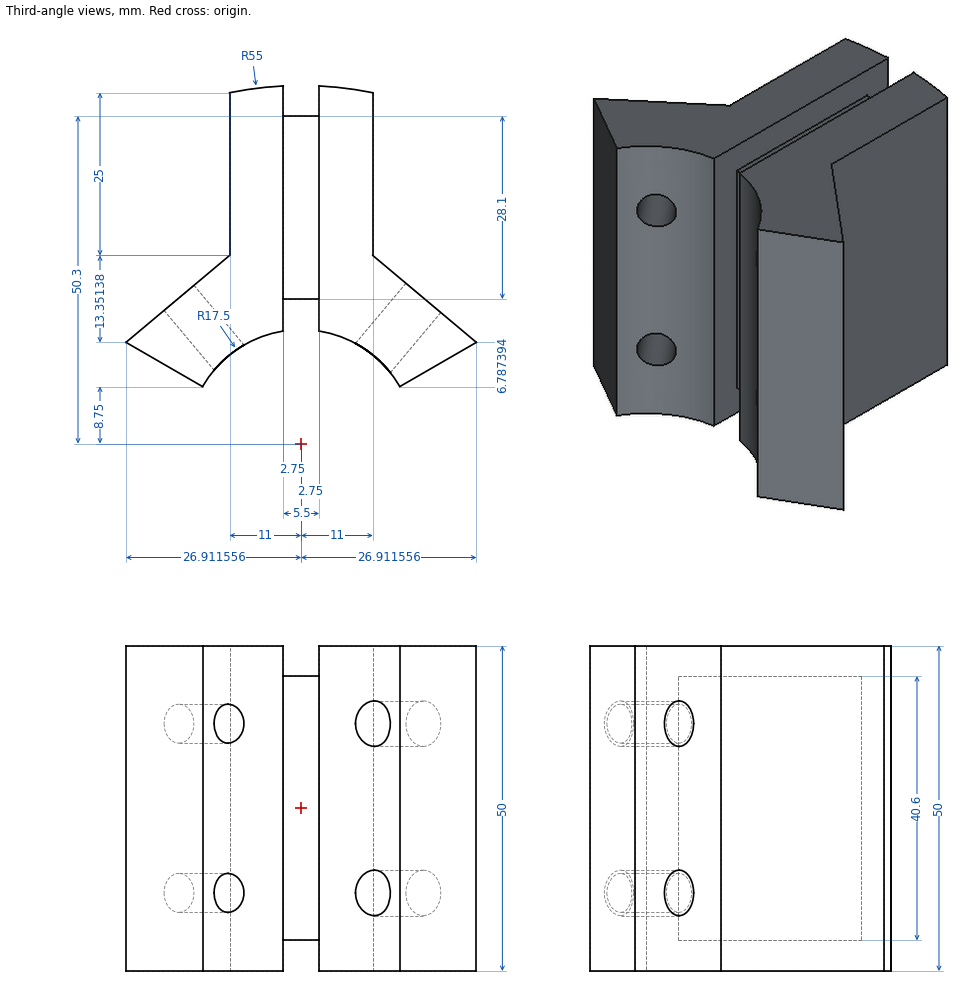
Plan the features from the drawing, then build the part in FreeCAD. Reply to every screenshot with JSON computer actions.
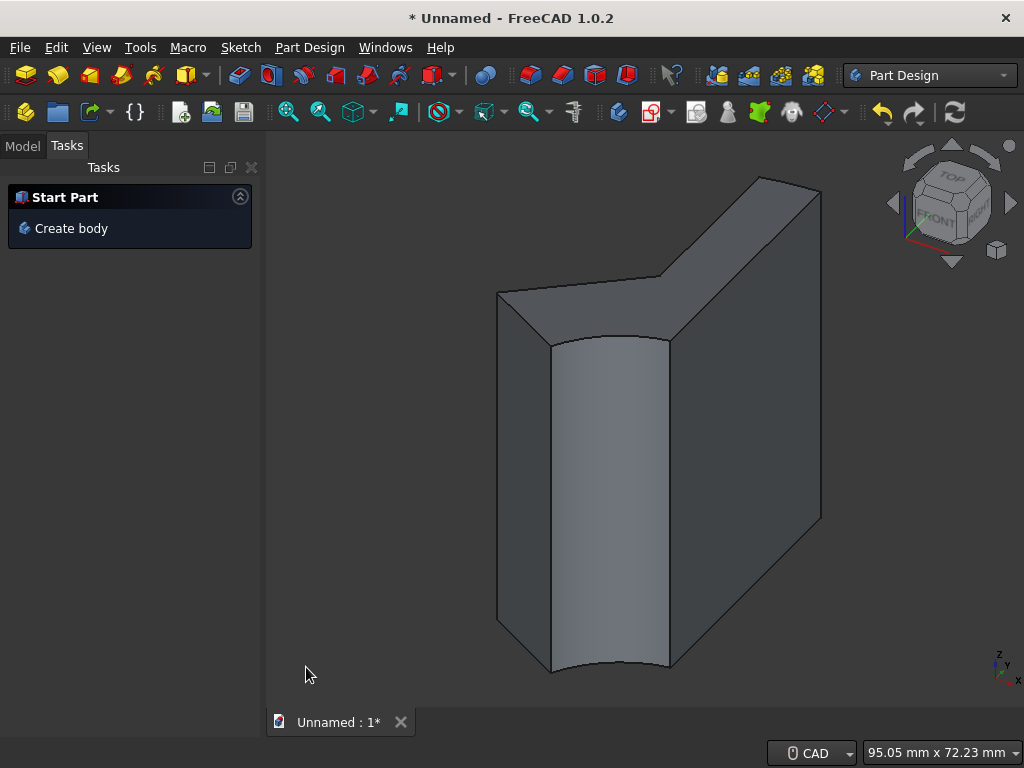
{"action": "left_click", "coordinate": [652, 112]}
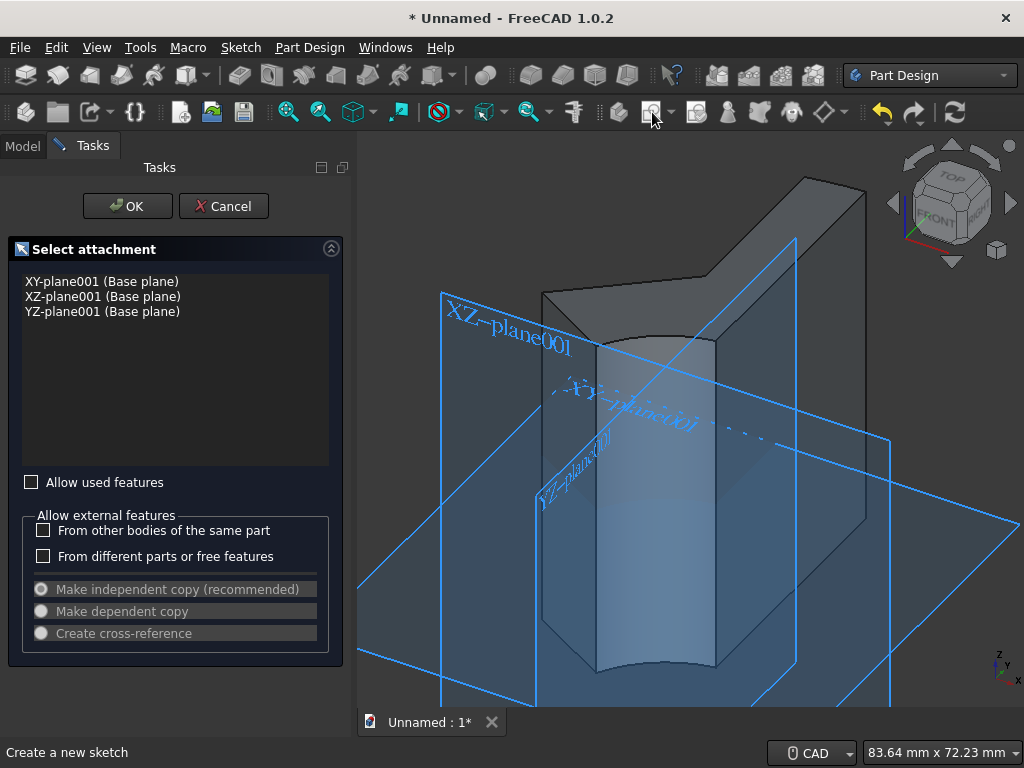
{"action": "left_click", "coordinate": [82, 282]}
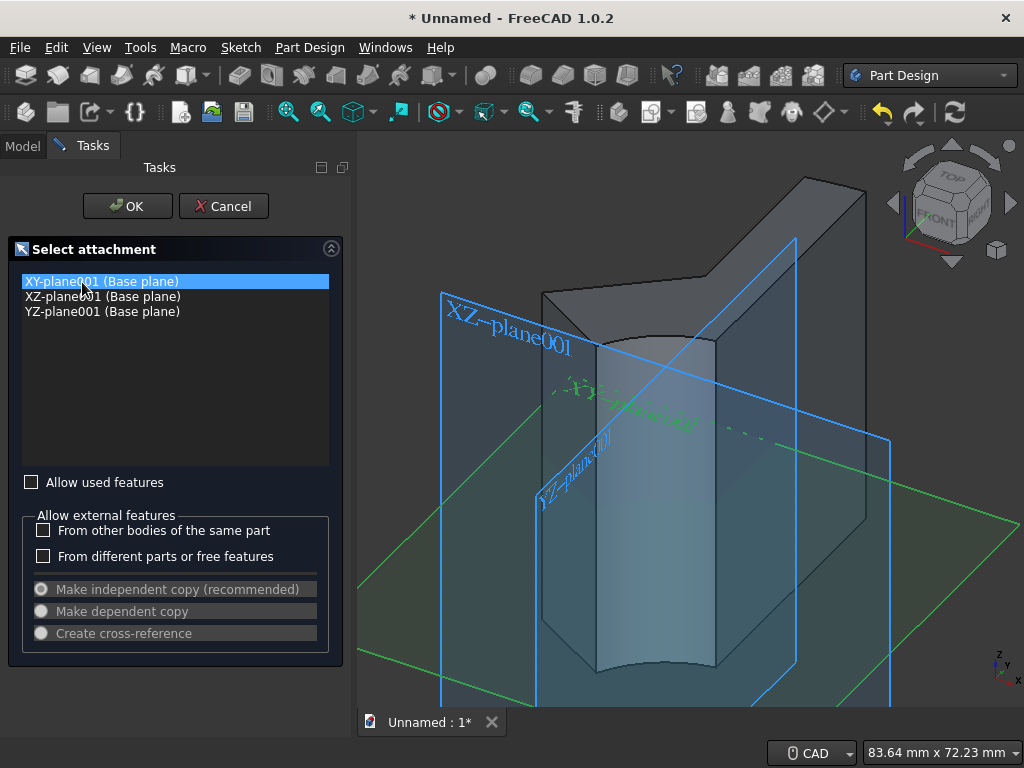
{"action": "left_click", "coordinate": [128, 206]}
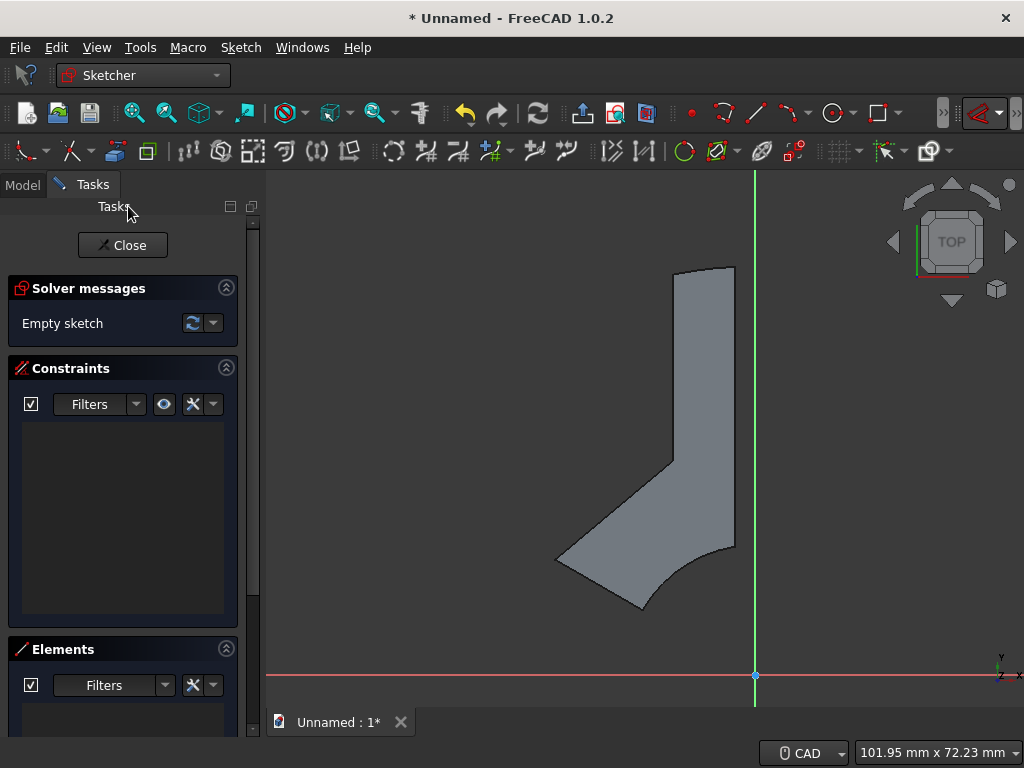
{"action": "scroll", "coordinate": [294, 372], "scroll_direction": "down", "scroll_amount": 2}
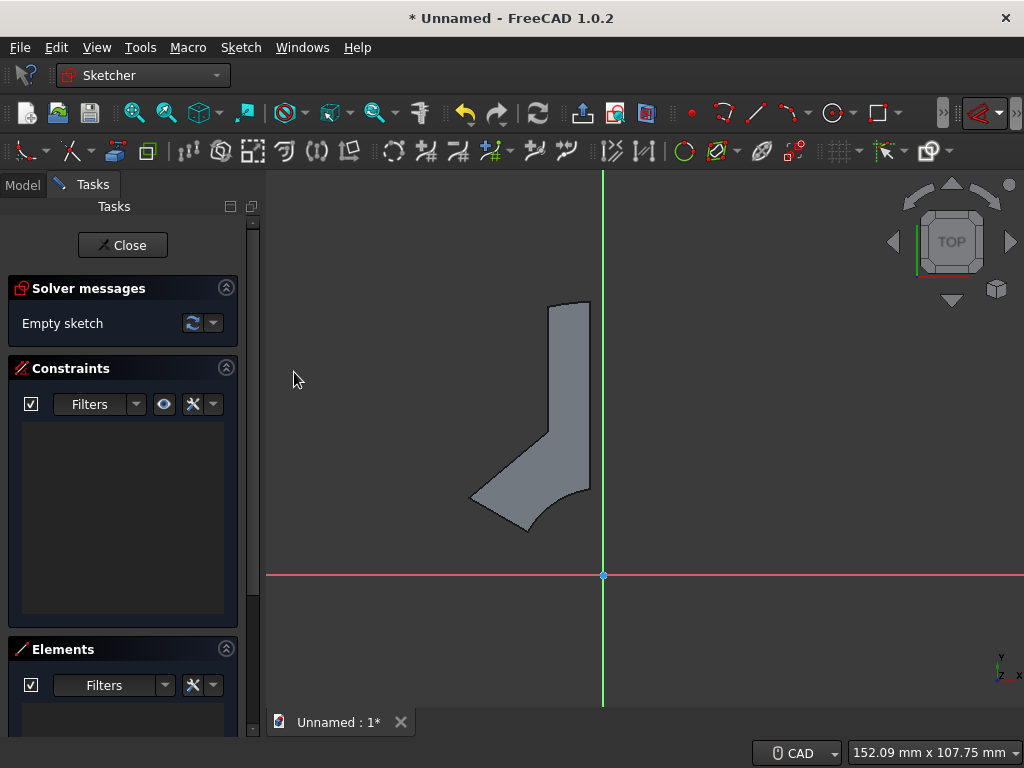
{"action": "left_click", "coordinate": [756, 114]}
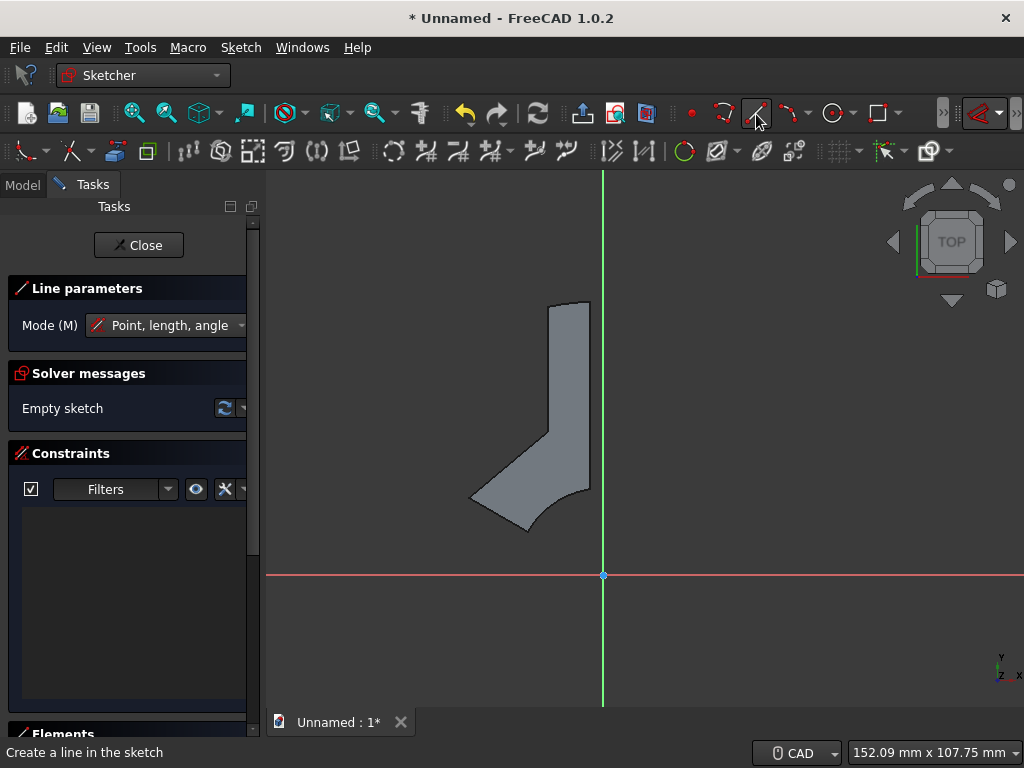
{"action": "left_click", "coordinate": [617, 302]}
{"action": "left_click", "coordinate": [617, 489]}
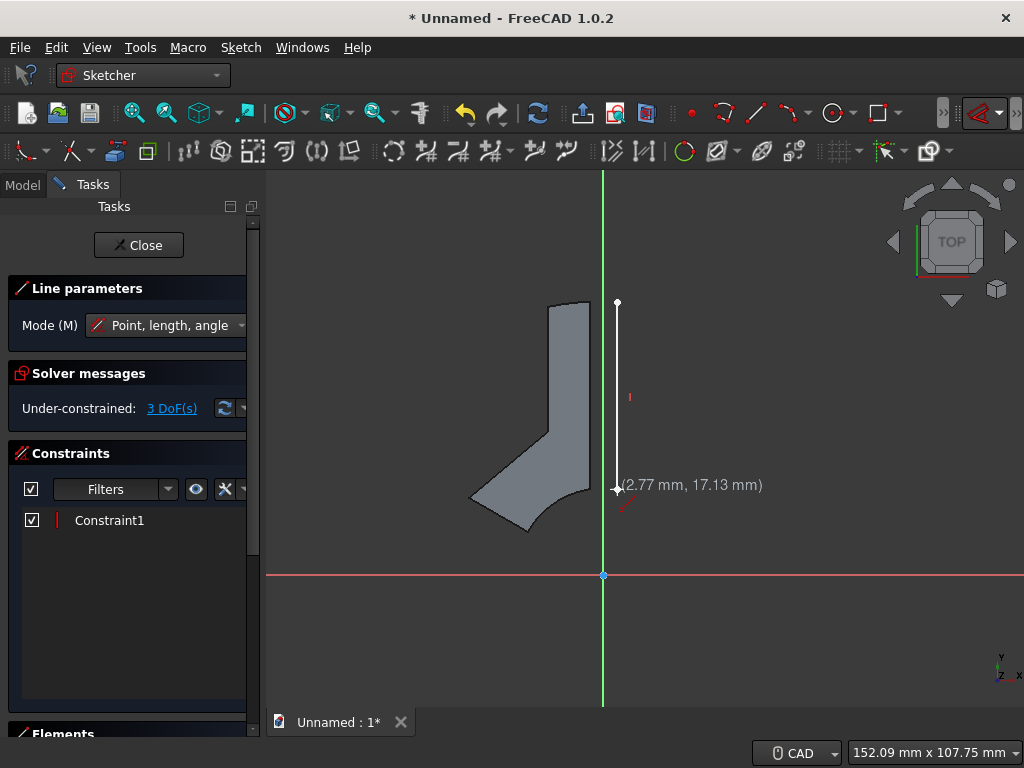
{"action": "left_click", "coordinate": [724, 114]}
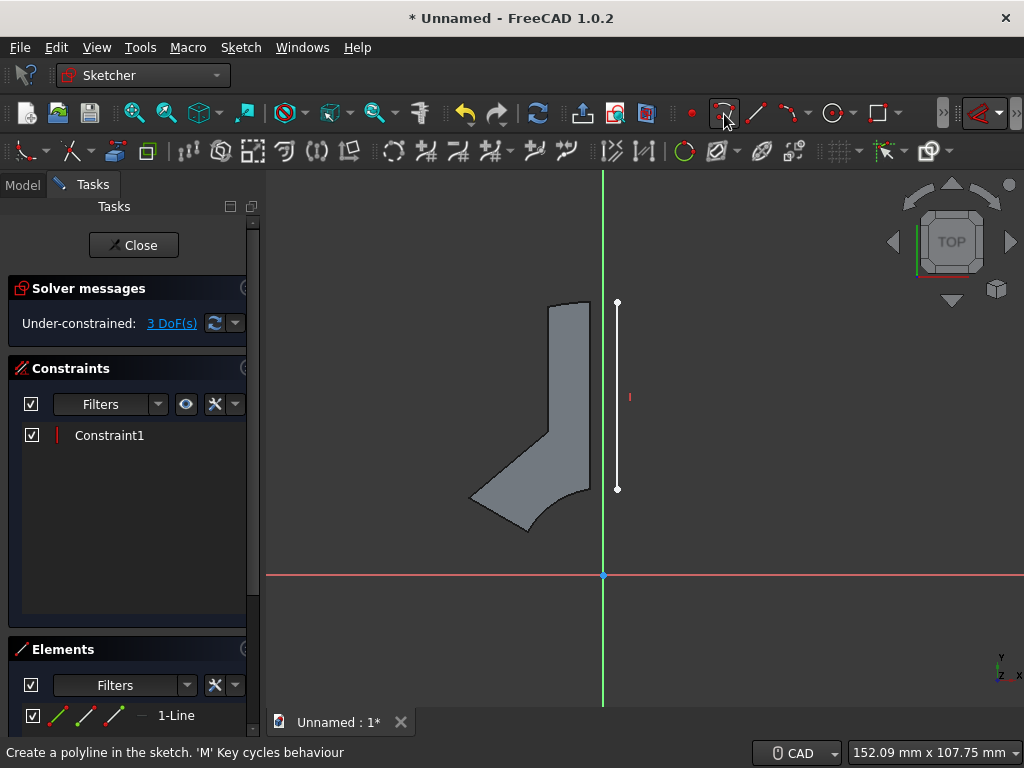
{"action": "left_click", "coordinate": [679, 532]}
{"action": "left_click", "coordinate": [737, 498]}
{"action": "left_click", "coordinate": [658, 431]}
{"action": "left_click", "coordinate": [658, 307]}
{"action": "right_click", "coordinate": [658, 307]}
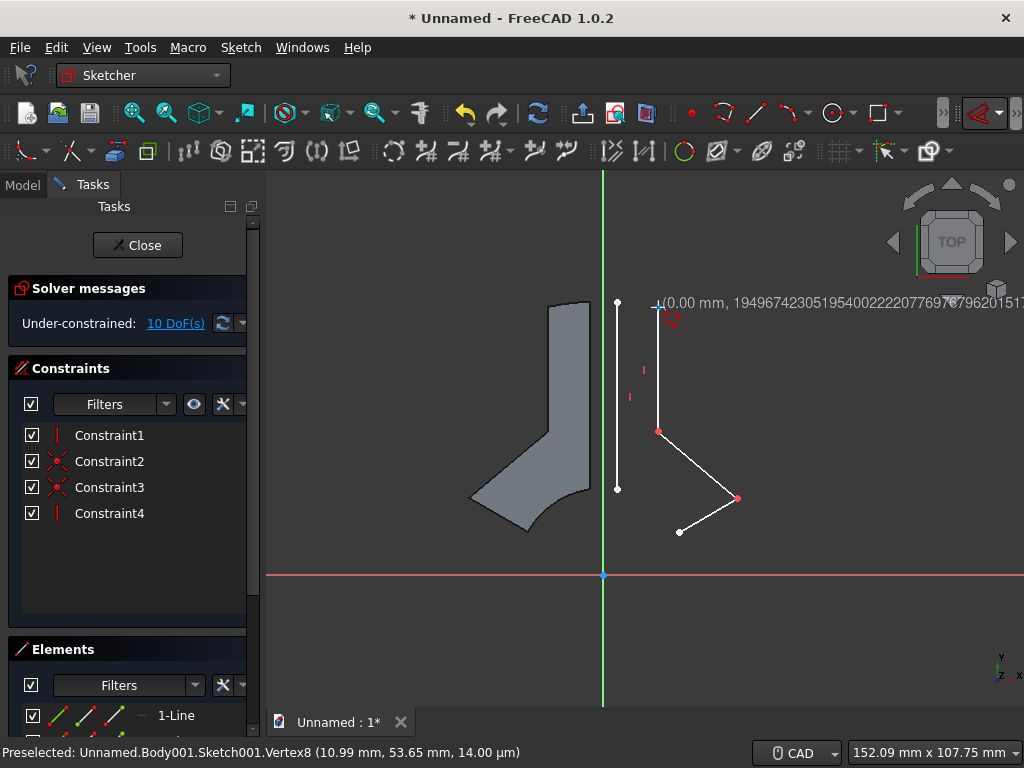
{"action": "left_click", "coordinate": [788, 114]}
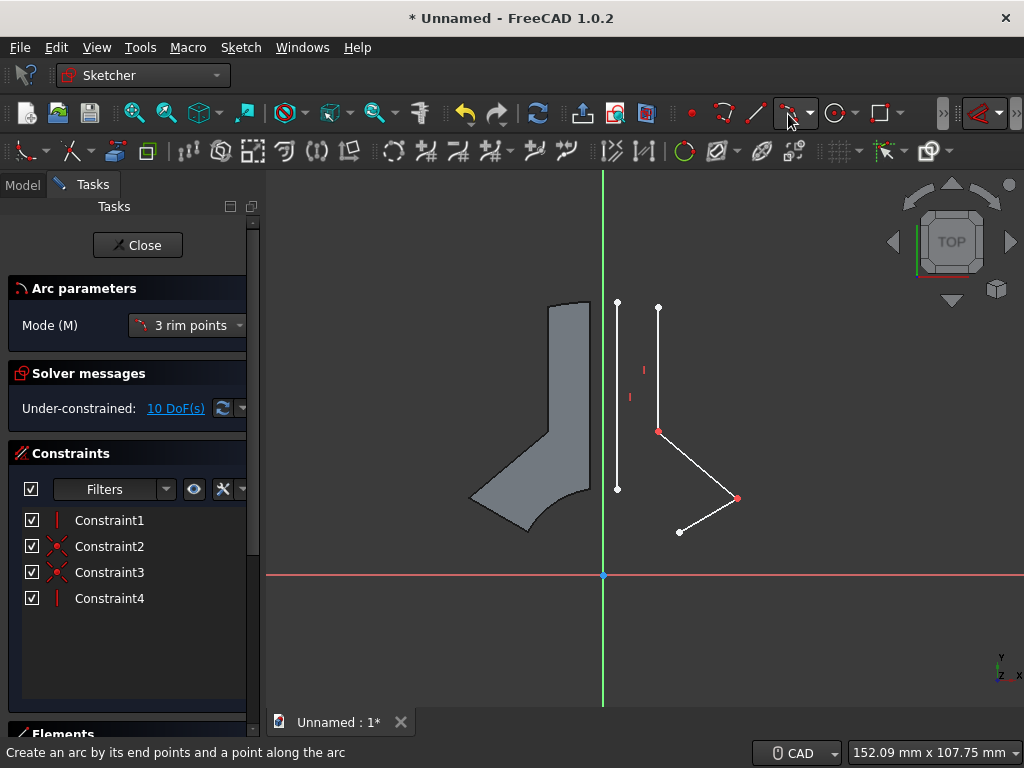
{"action": "left_click", "coordinate": [617, 490]}
{"action": "left_click", "coordinate": [679, 533]}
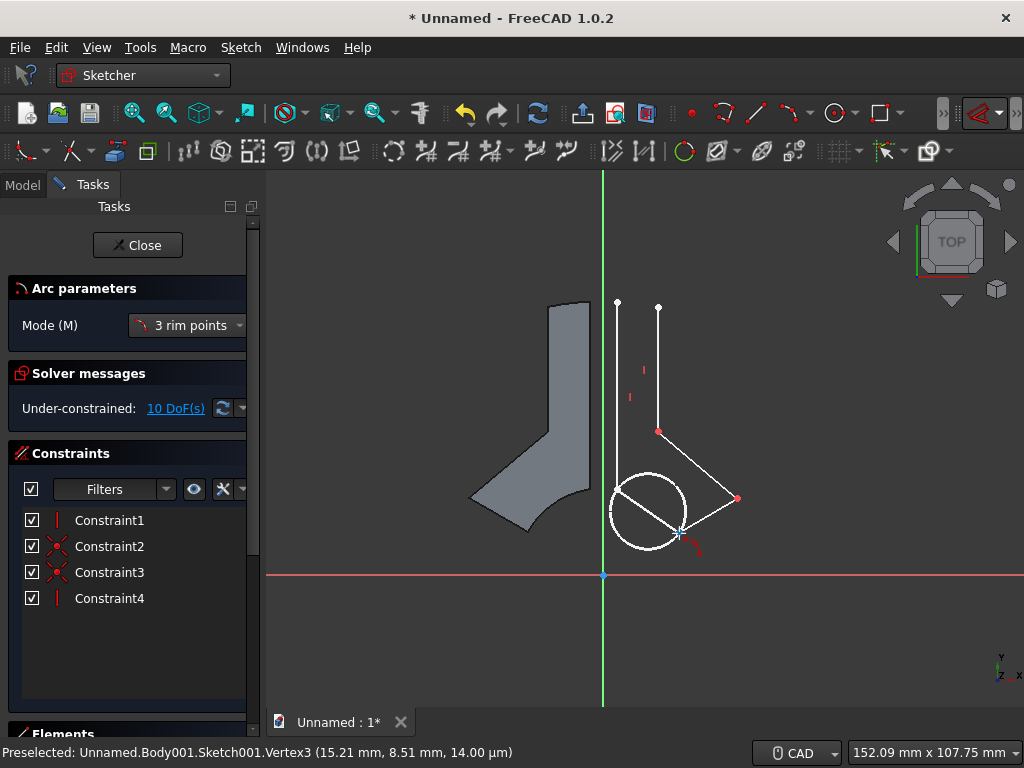
{"action": "scroll", "coordinate": [653, 504], "scroll_direction": "up", "scroll_amount": 4}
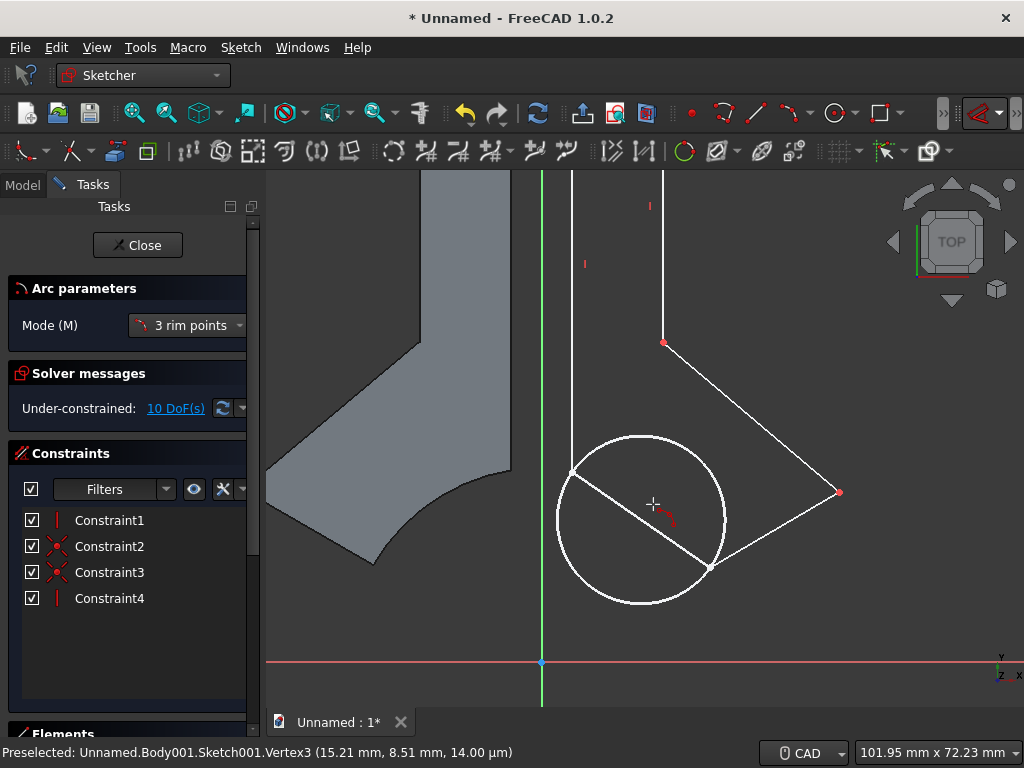
{"action": "left_click", "coordinate": [652, 502]}